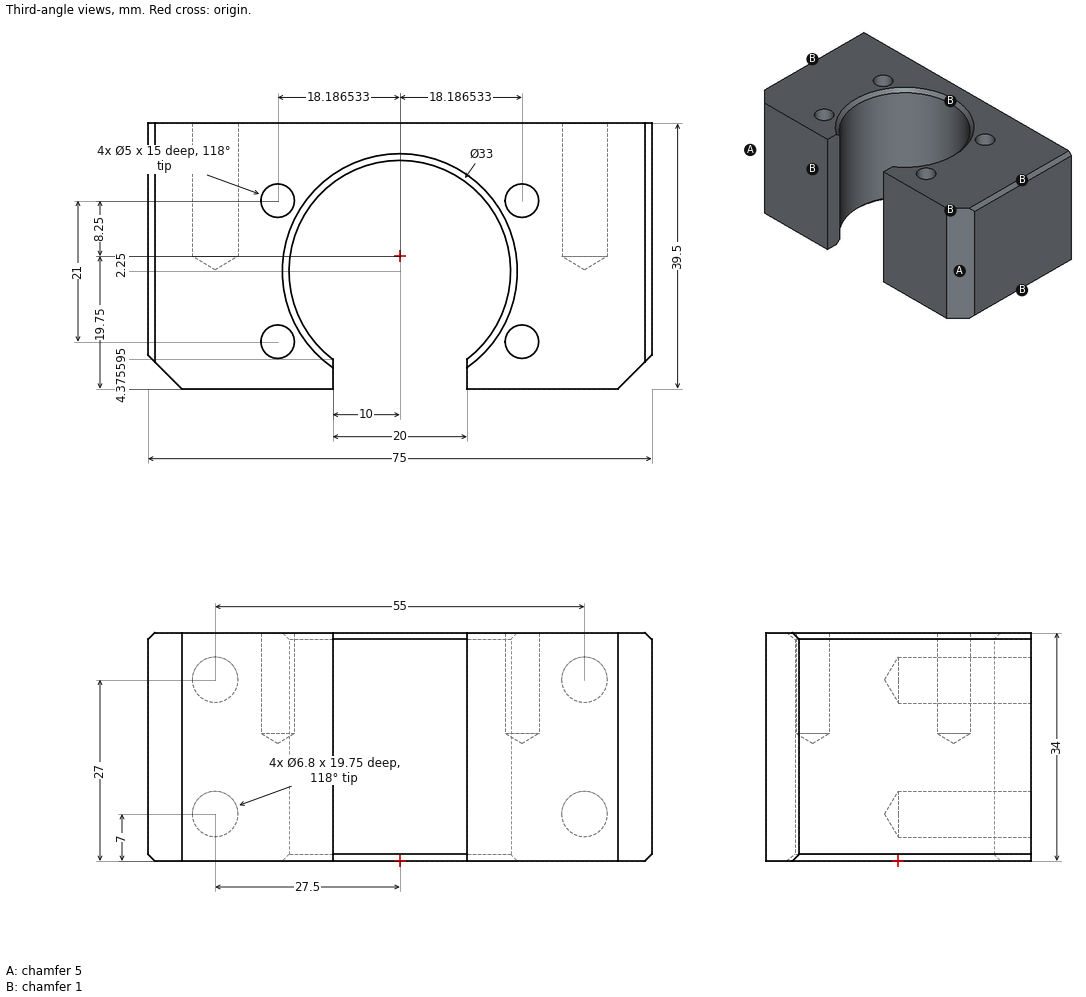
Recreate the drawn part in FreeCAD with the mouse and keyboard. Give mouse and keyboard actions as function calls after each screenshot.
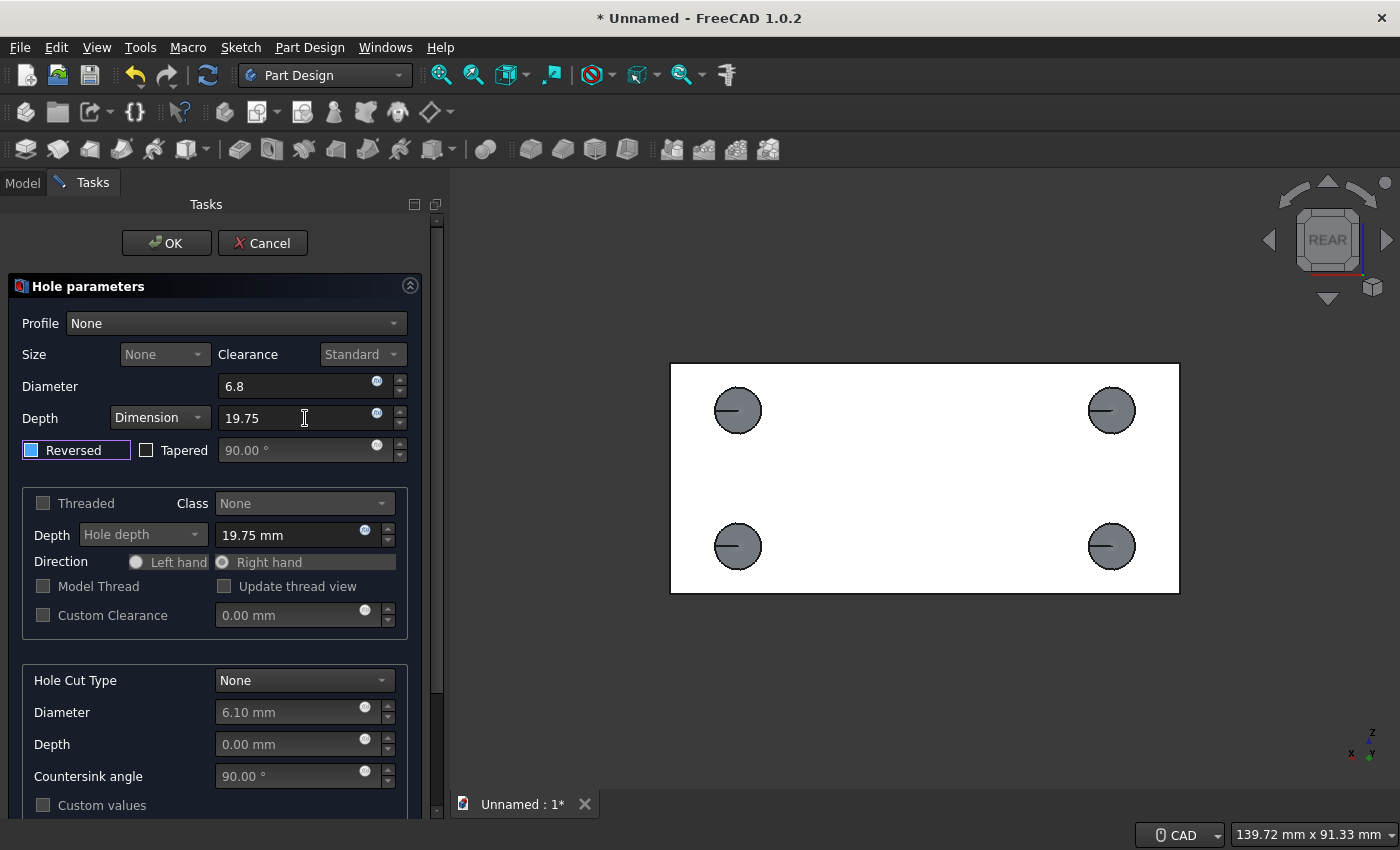
click(167, 243)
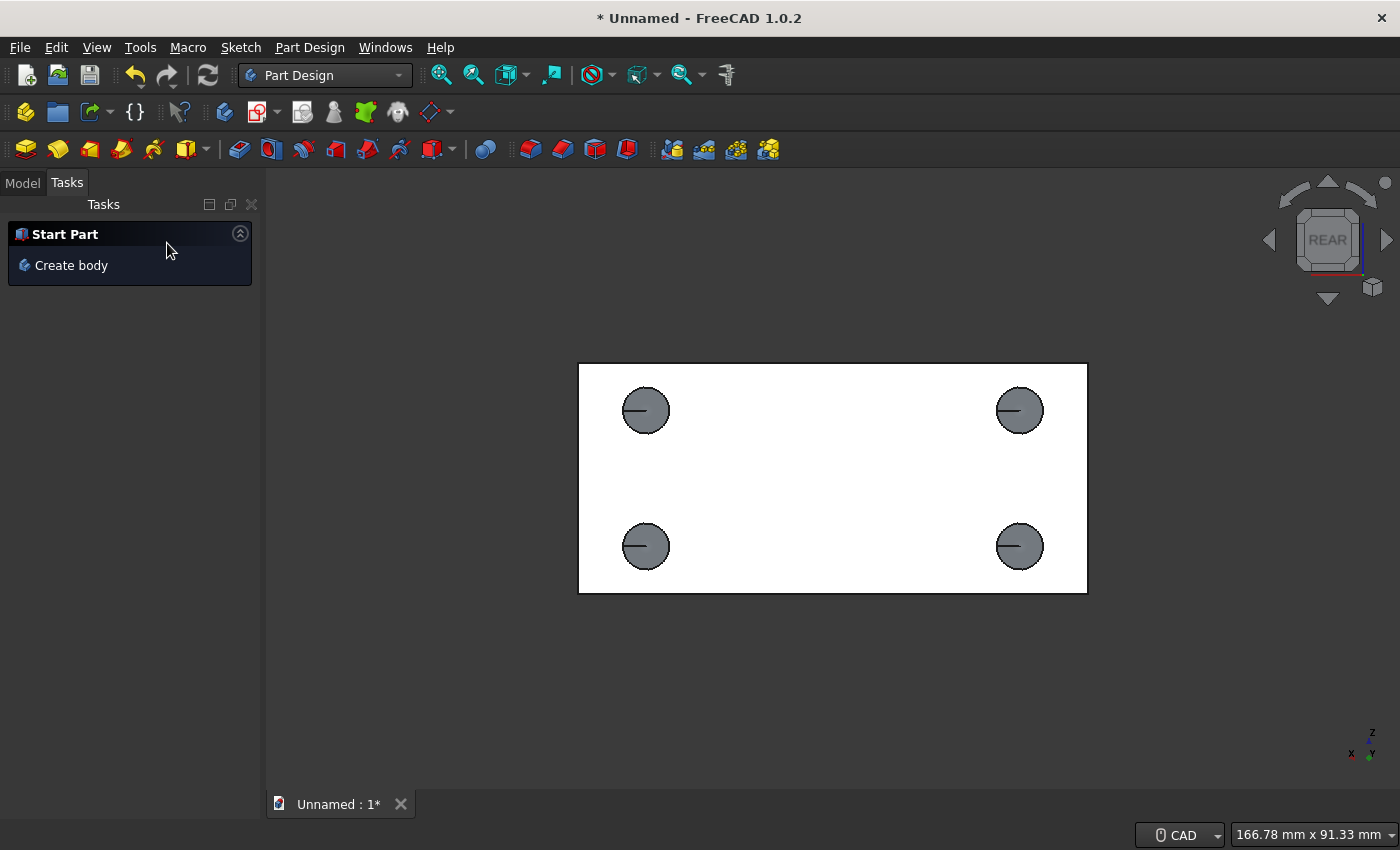
click(442, 76)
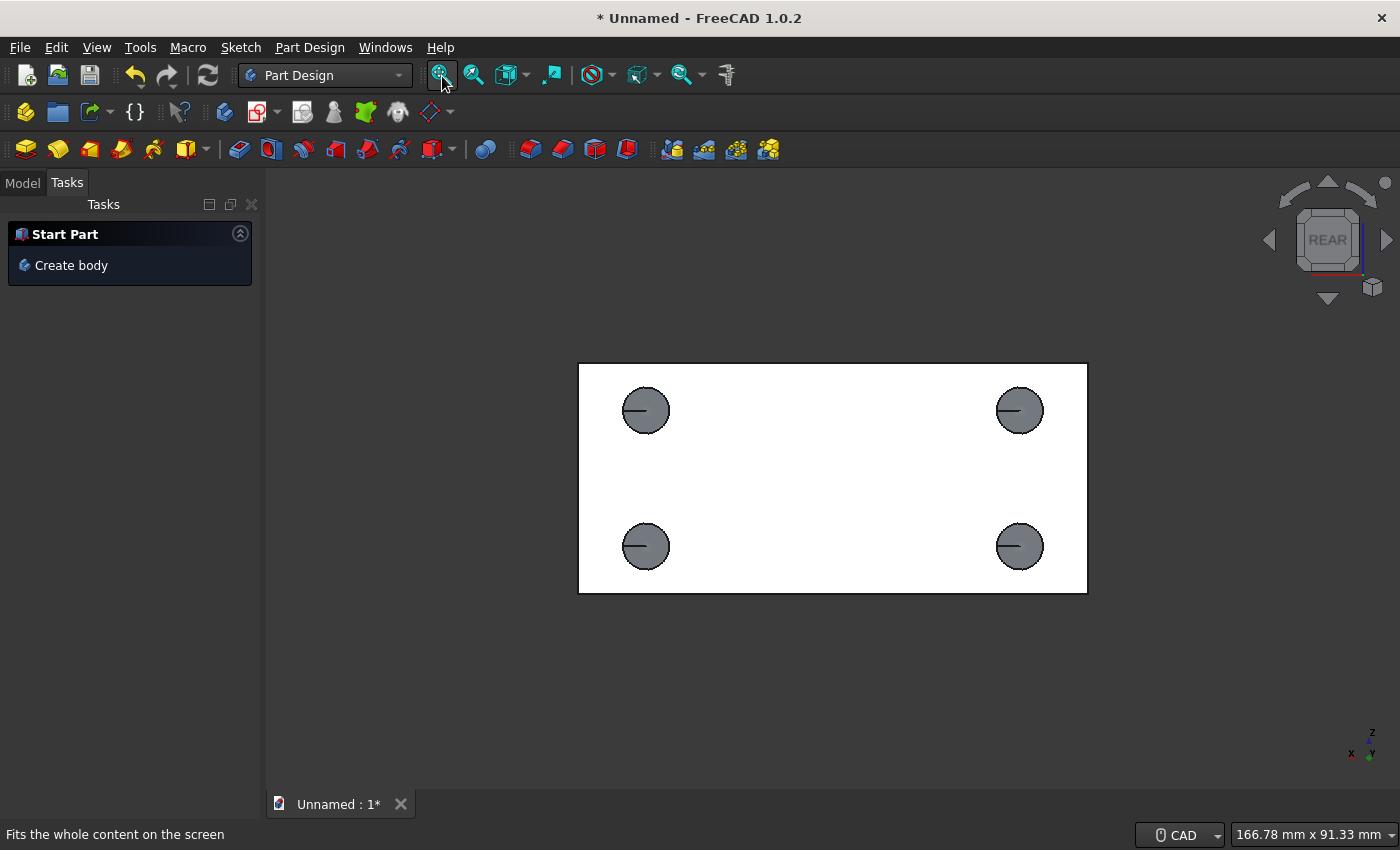
key(0)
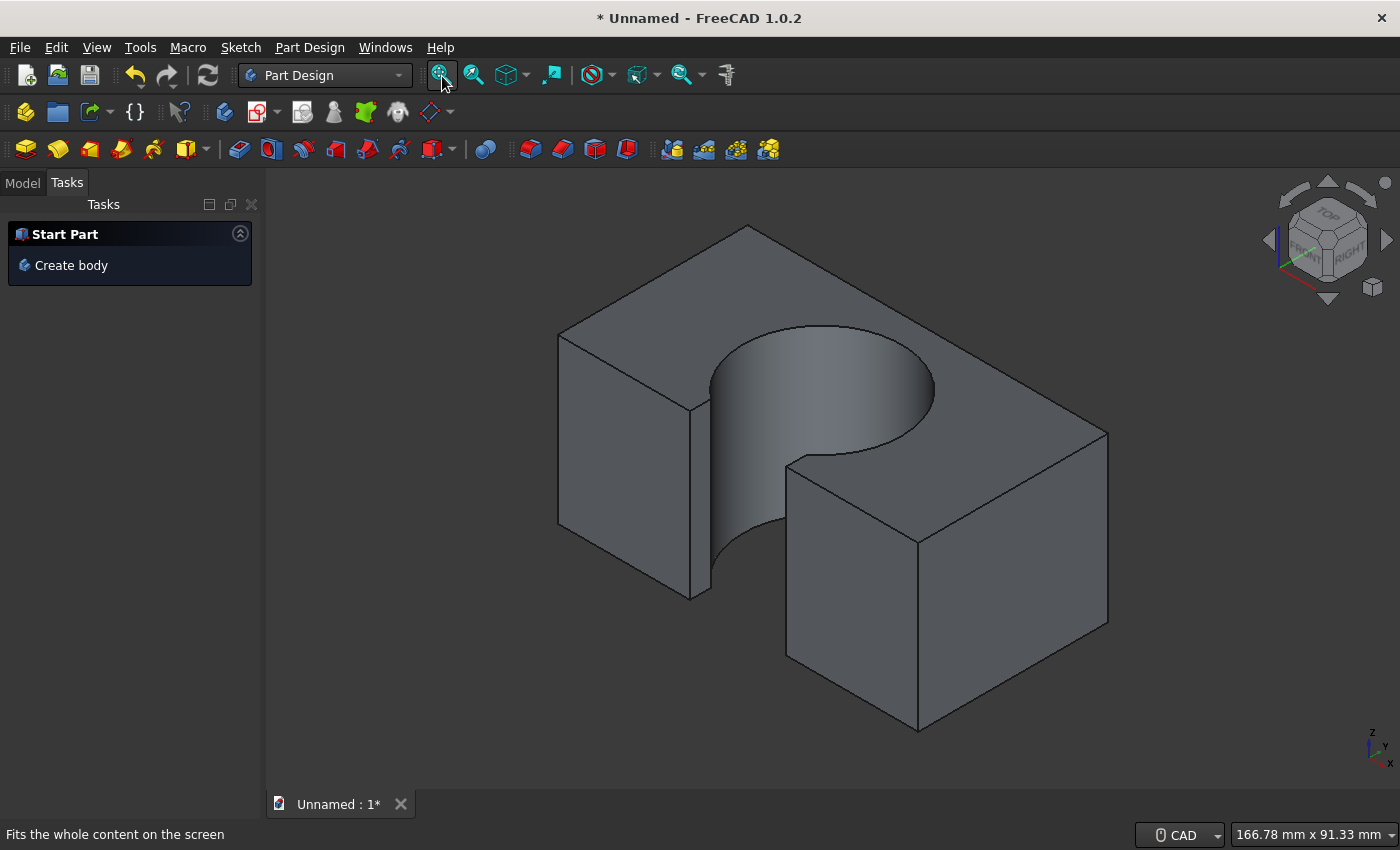
click(918, 636)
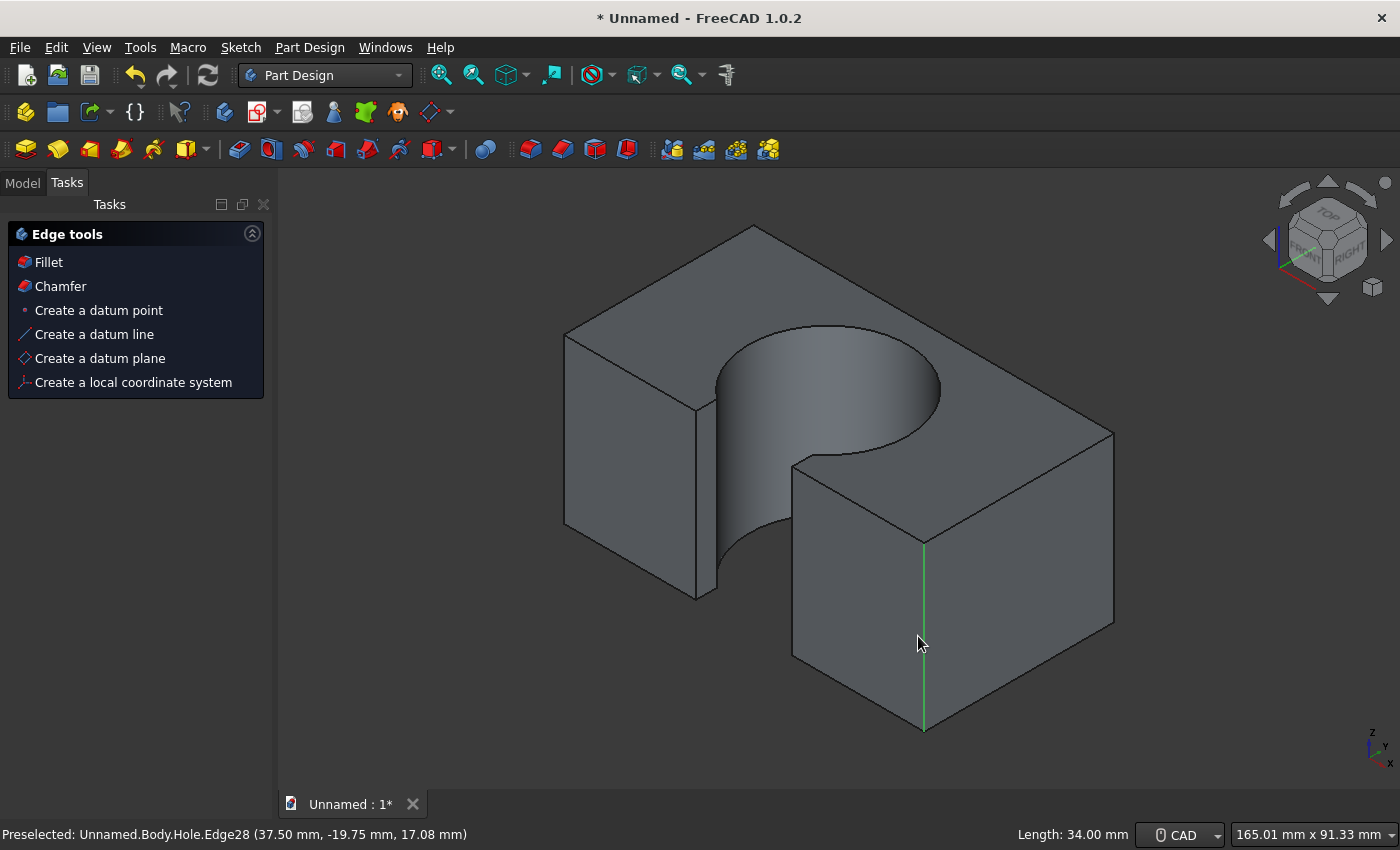
key(2)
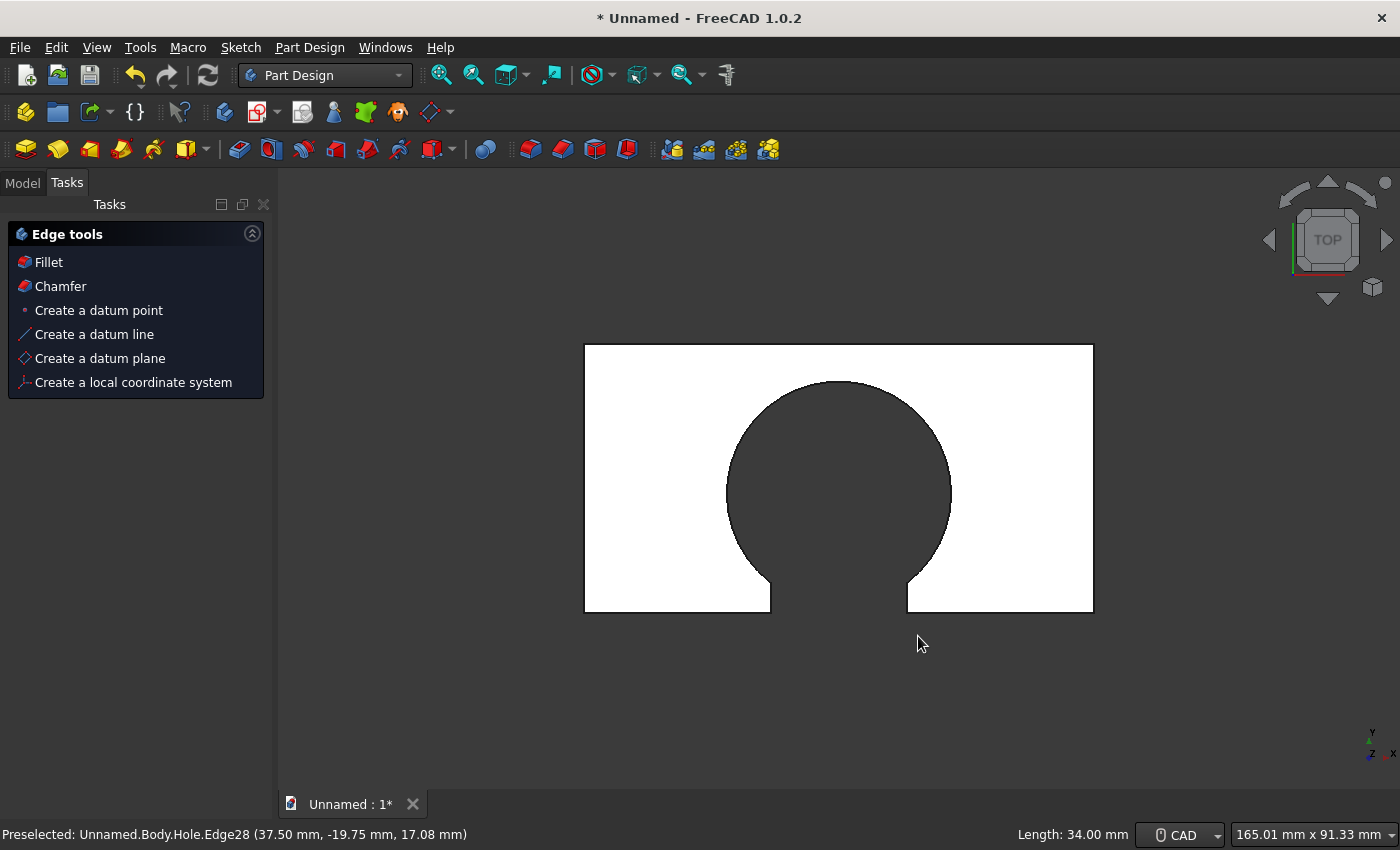
key(1)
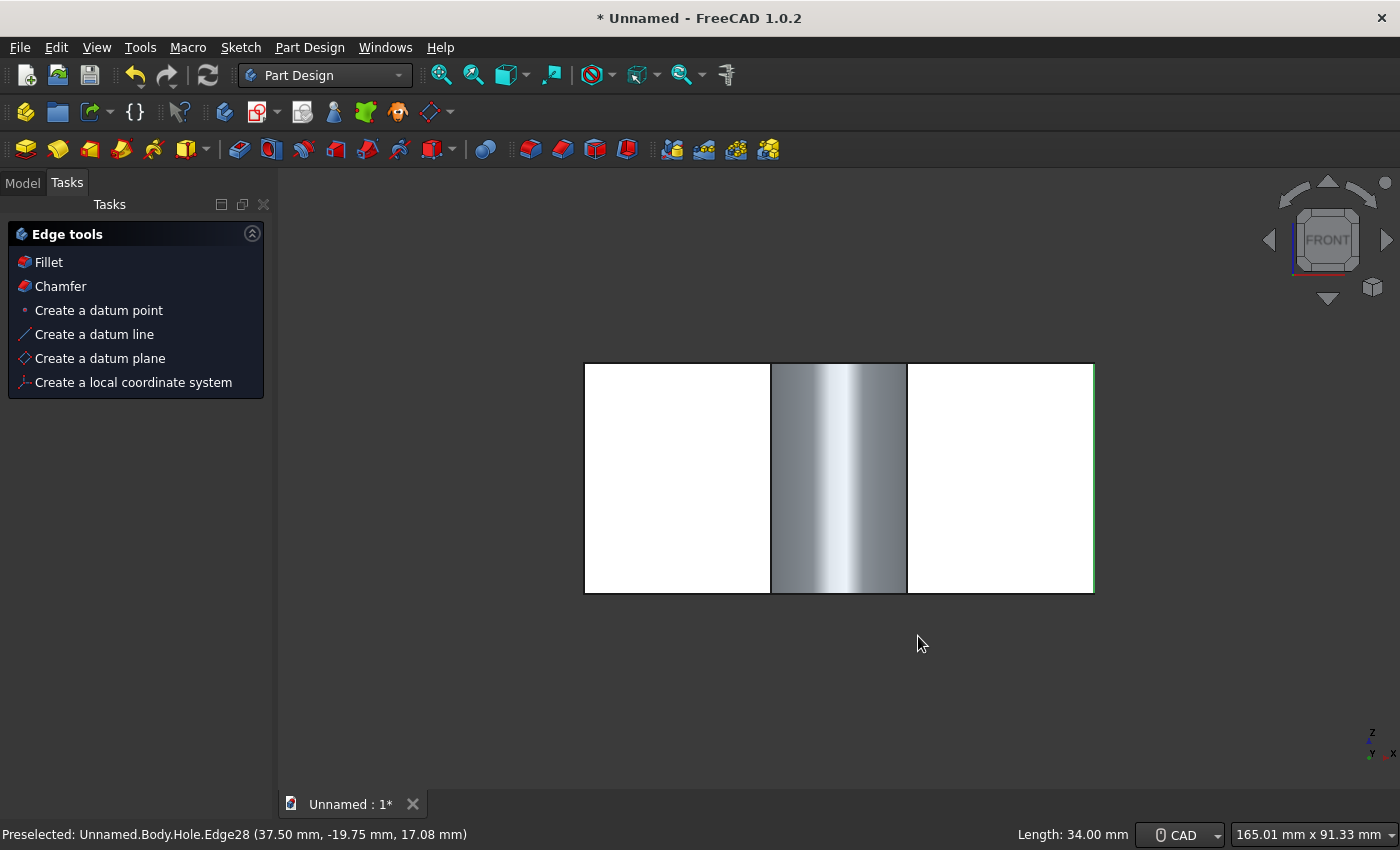
click(584, 477, ctrl)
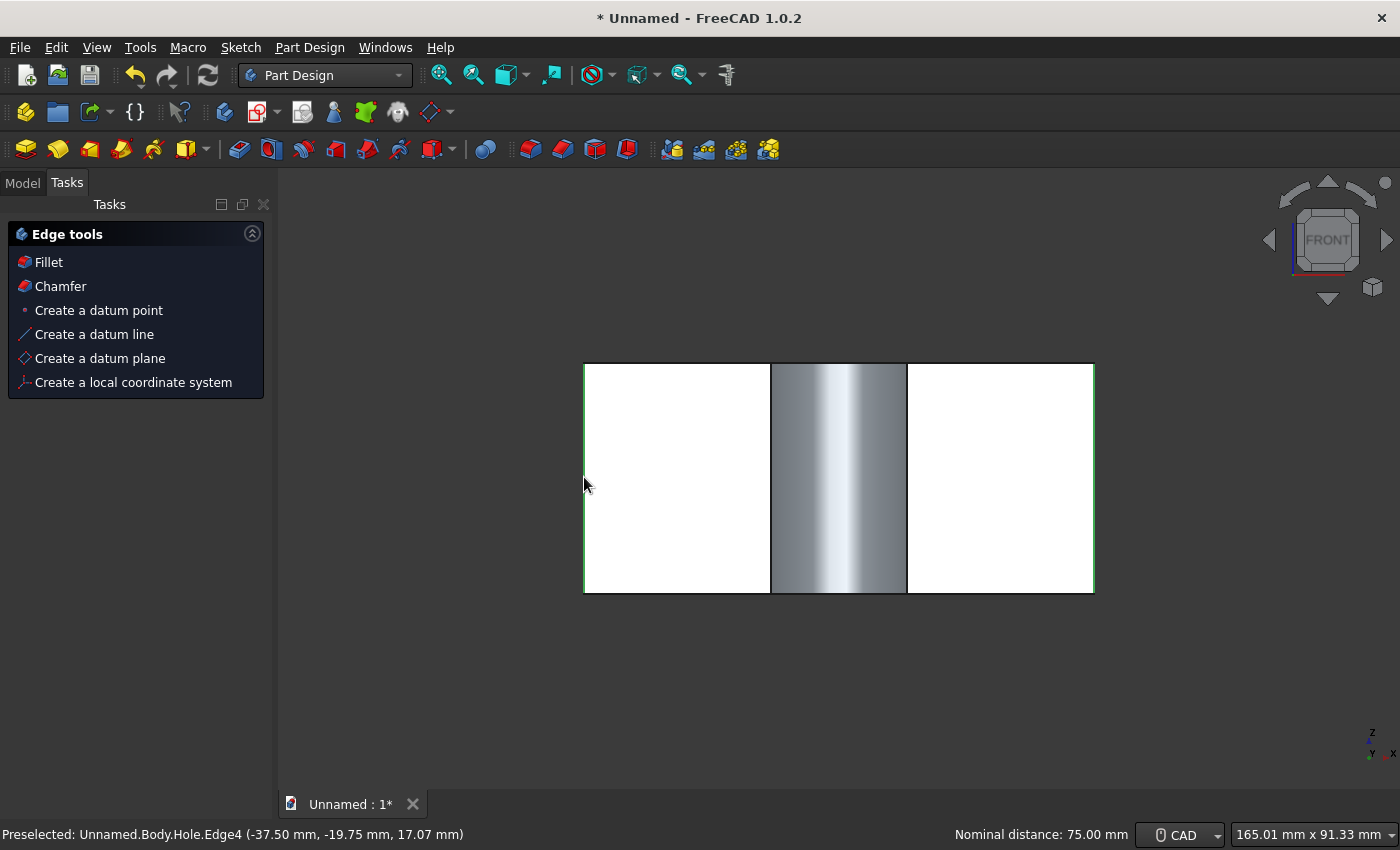
click(564, 150)